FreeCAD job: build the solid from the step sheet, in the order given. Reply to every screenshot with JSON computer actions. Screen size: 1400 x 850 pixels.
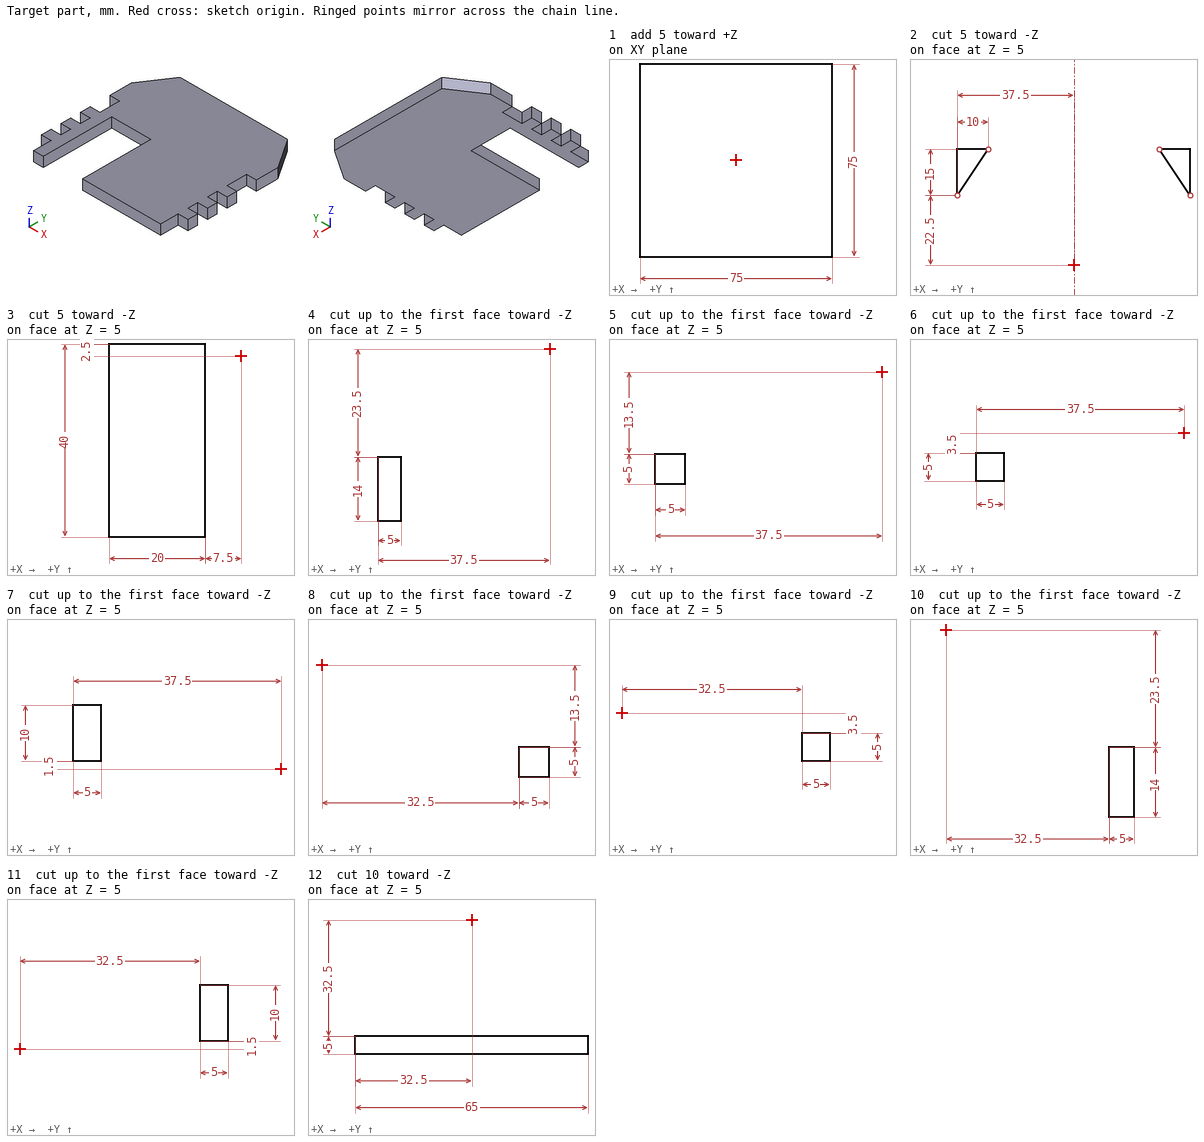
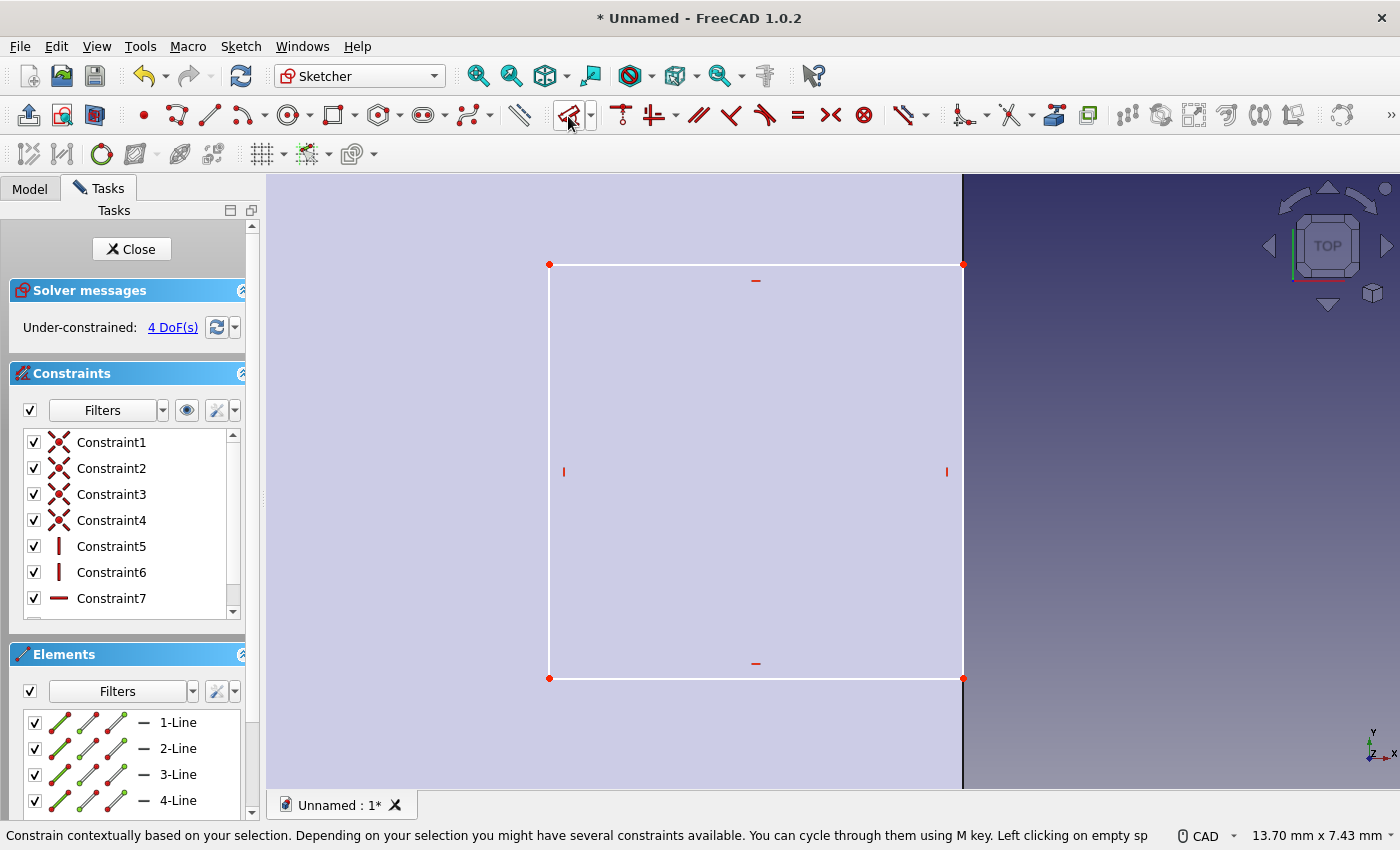
{"action": "left_click", "coordinate": [549, 389]}
{"action": "left_click", "coordinate": [515, 472]}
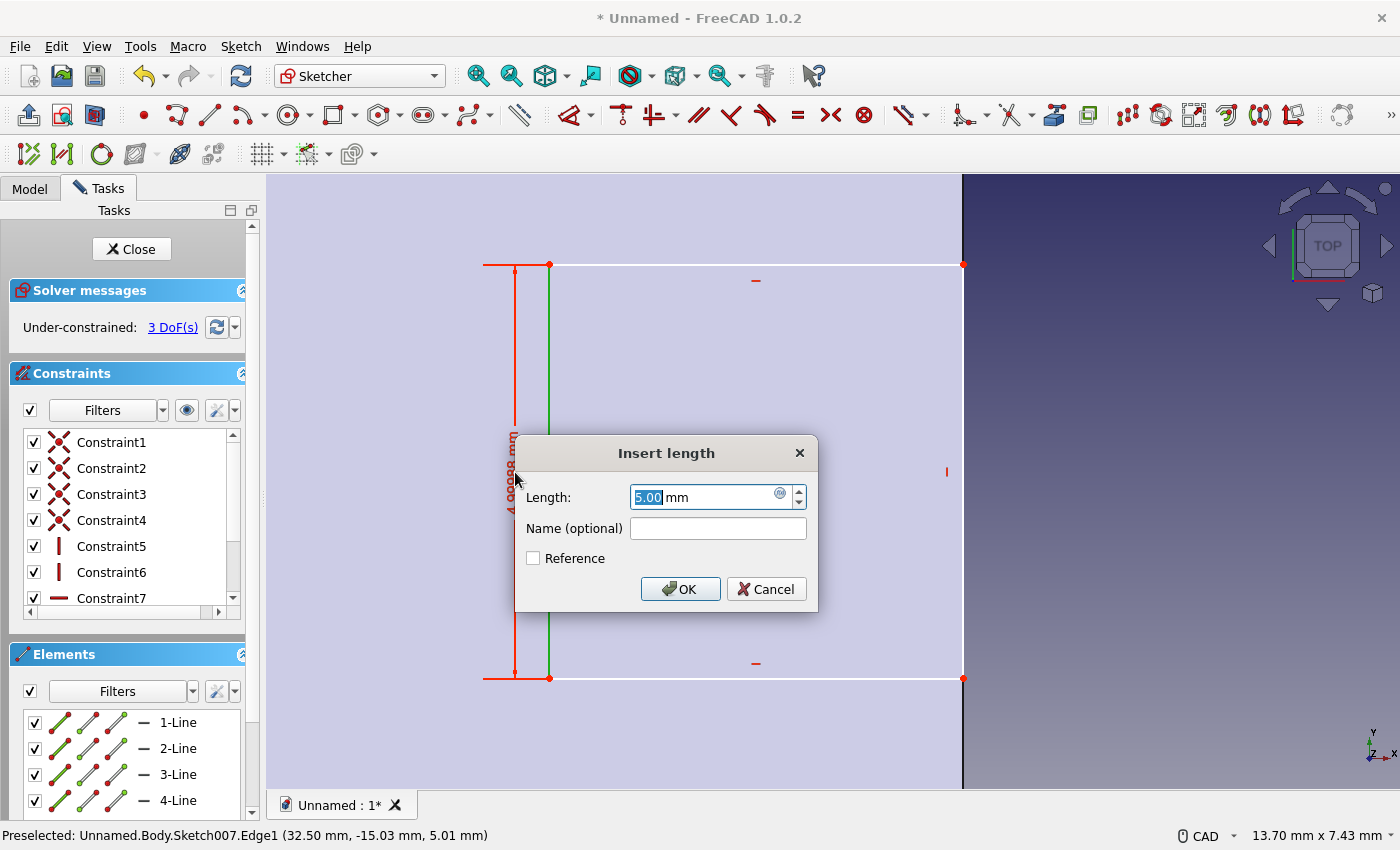
{"action": "type", "text": "5"}
{"action": "key", "text": "Return"}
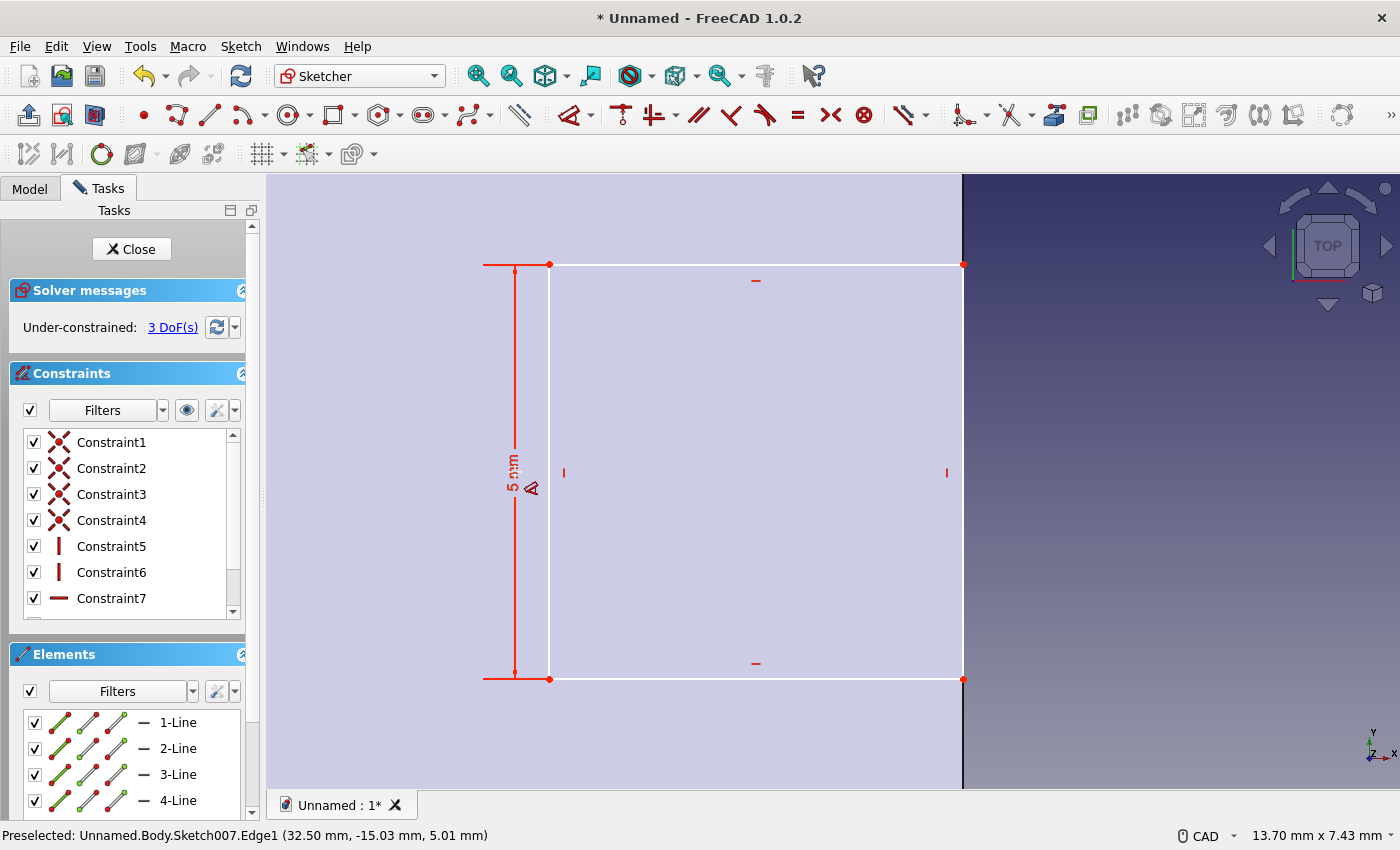
{"action": "left_click", "coordinate": [673, 679]}
{"action": "left_click", "coordinate": [756, 713]}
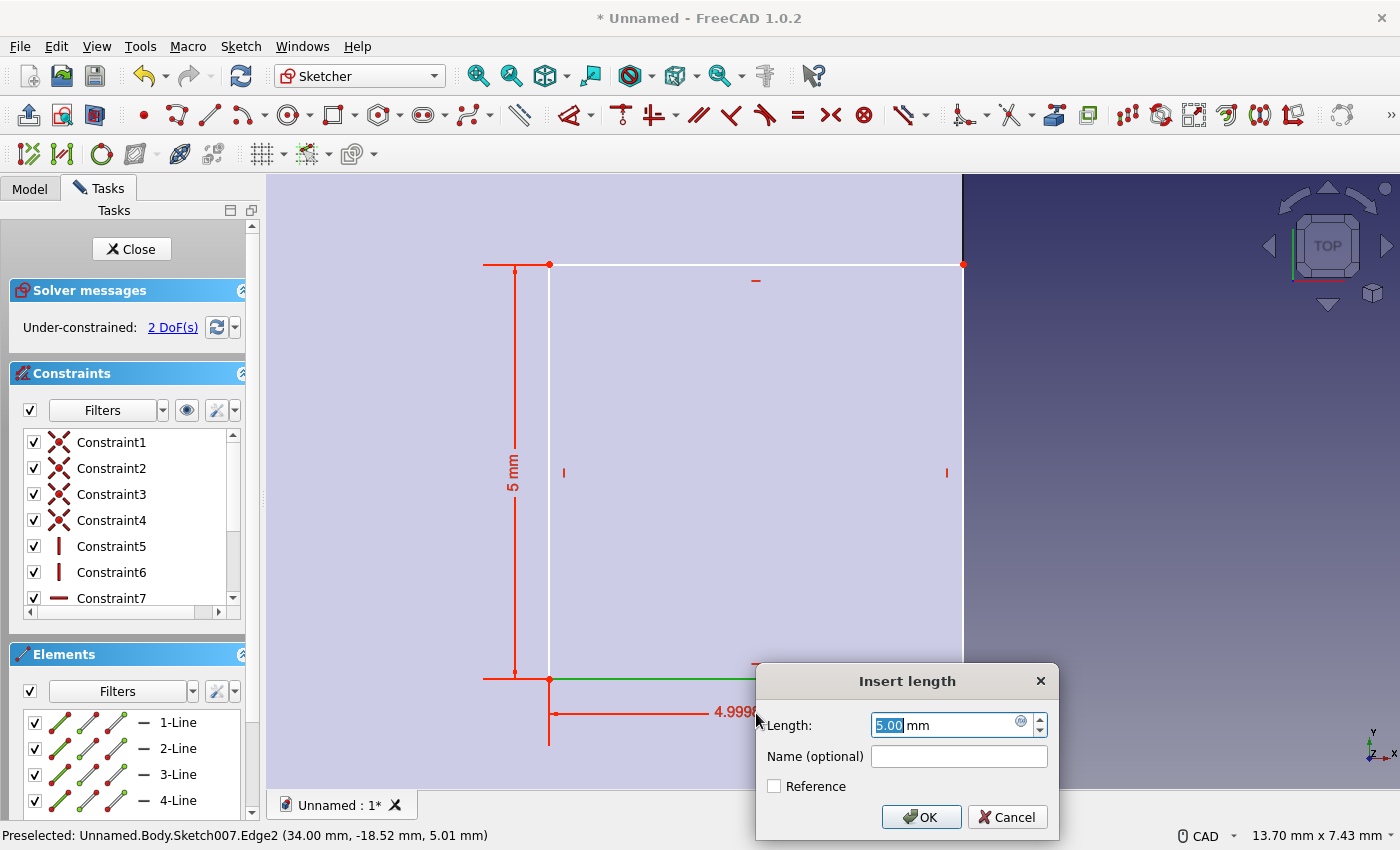
{"action": "type", "text": "5"}
{"action": "key", "text": "Return"}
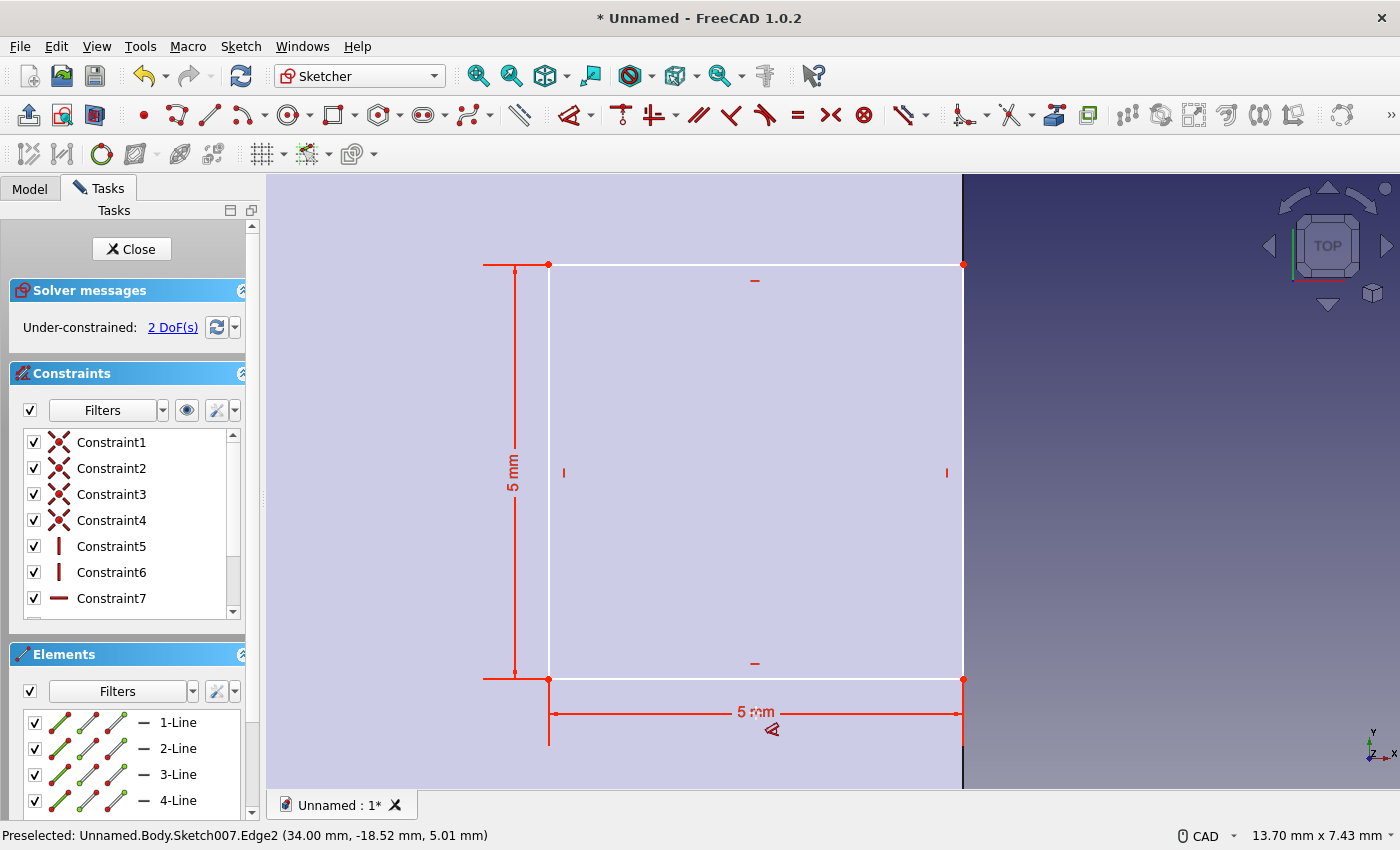
{"action": "left_click", "coordinate": [549, 265]}
{"action": "left_click", "coordinate": [421, 299]}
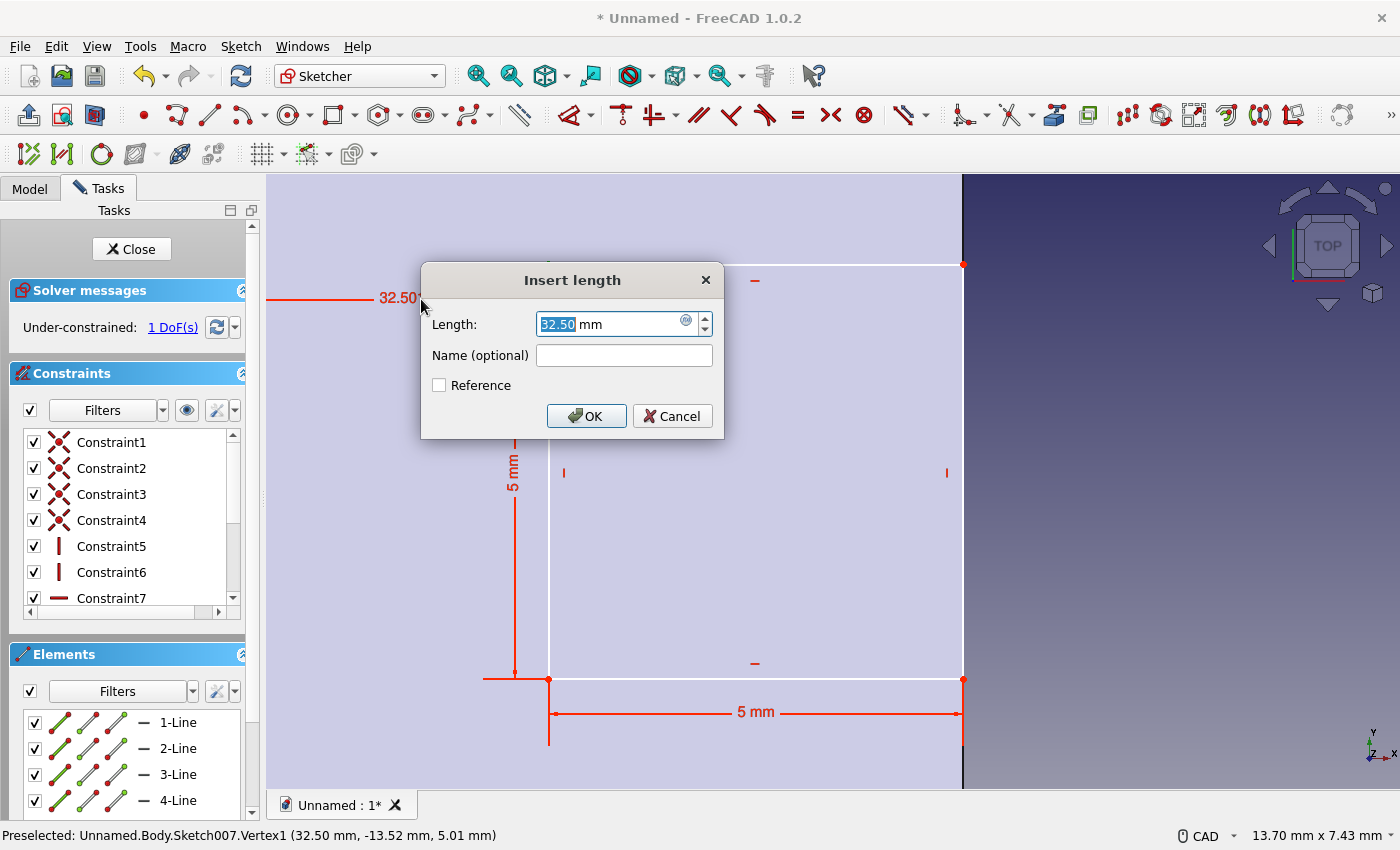
{"action": "type", "text": "32.5"}
{"action": "key", "text": "Return"}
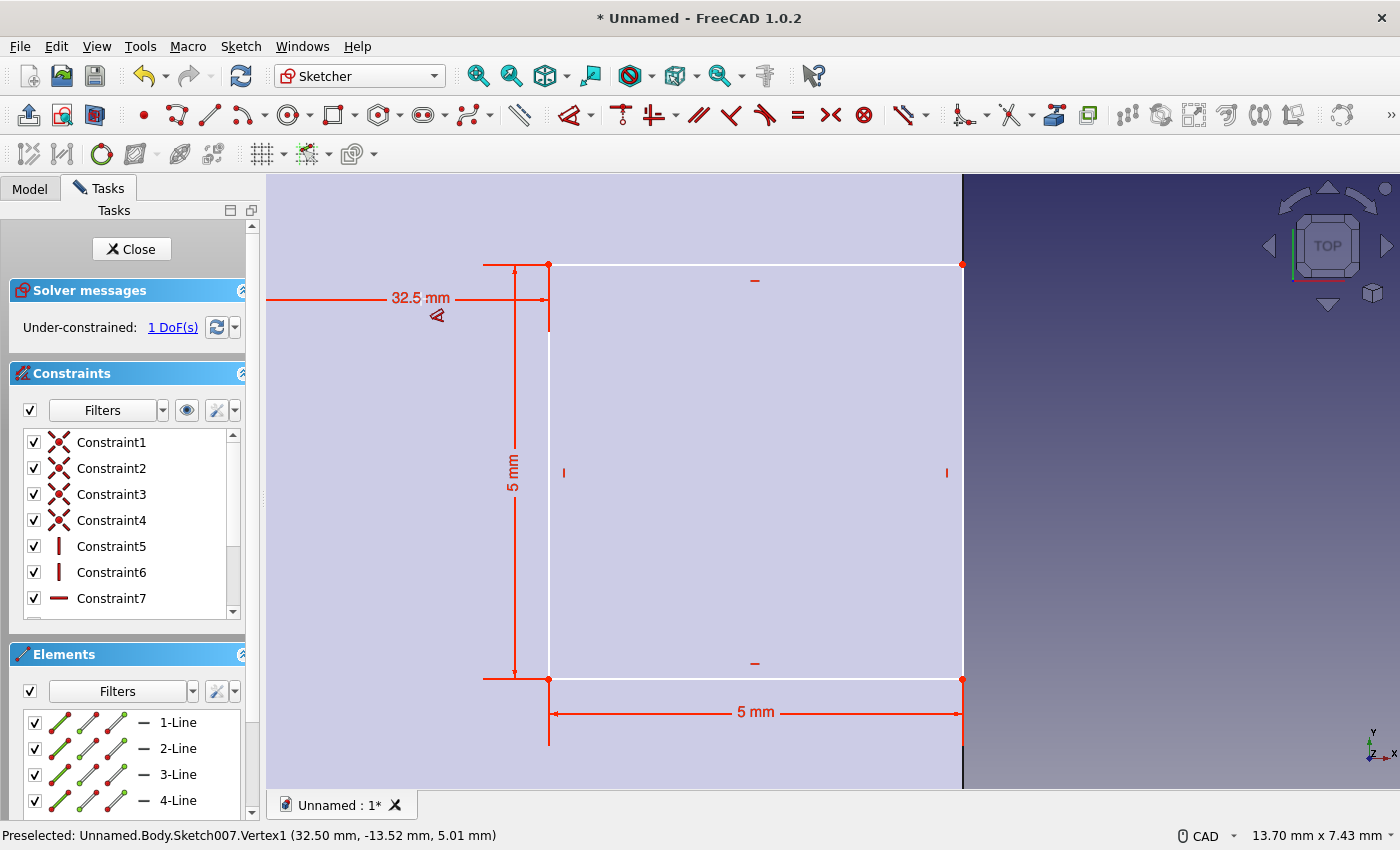
{"action": "left_click", "coordinate": [549, 265]}
{"action": "left_click", "coordinate": [583, 233]}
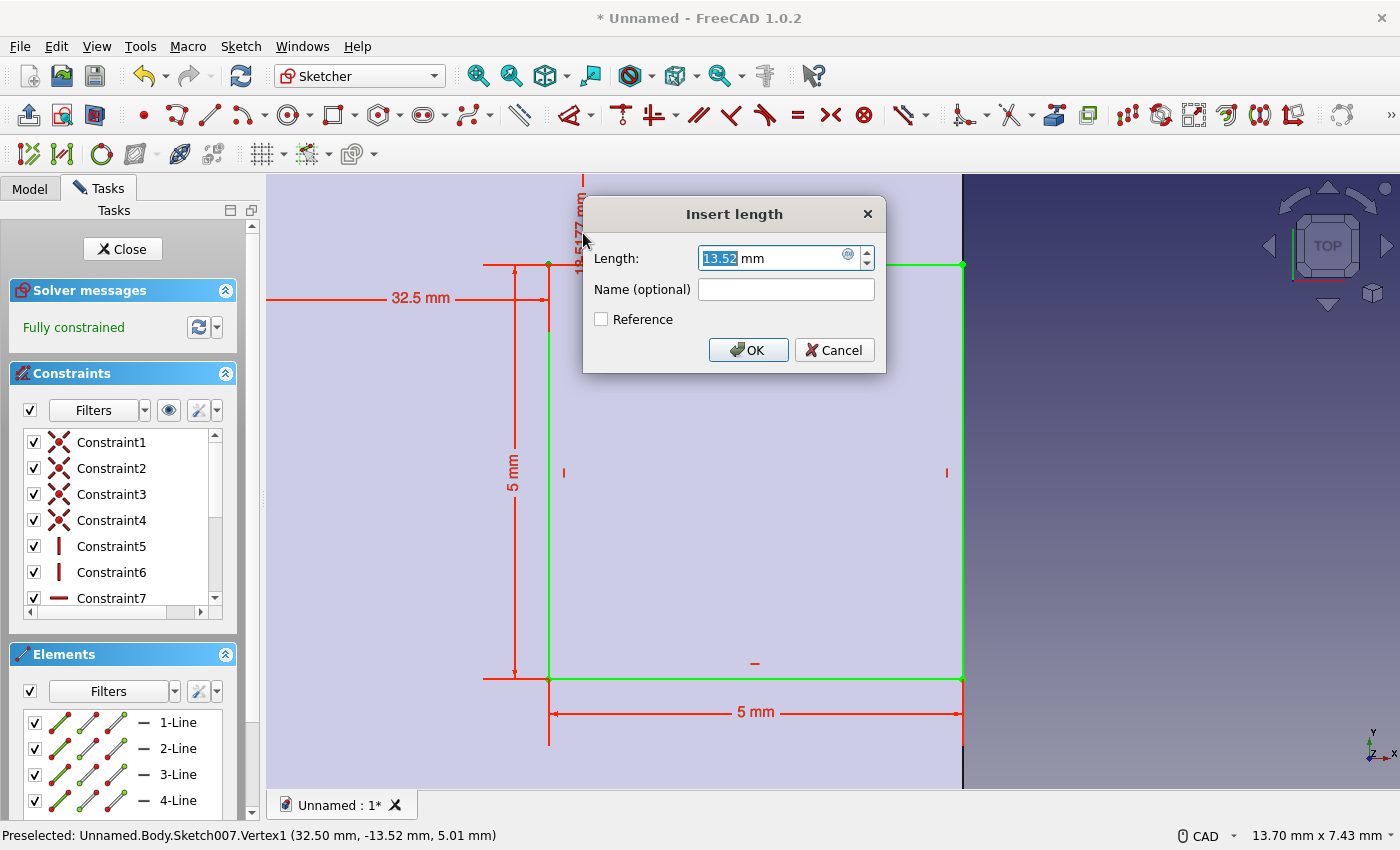
{"action": "type", "text": "13.5"}
{"action": "key", "text": "Return"}
{"action": "key", "text": "Escape"}